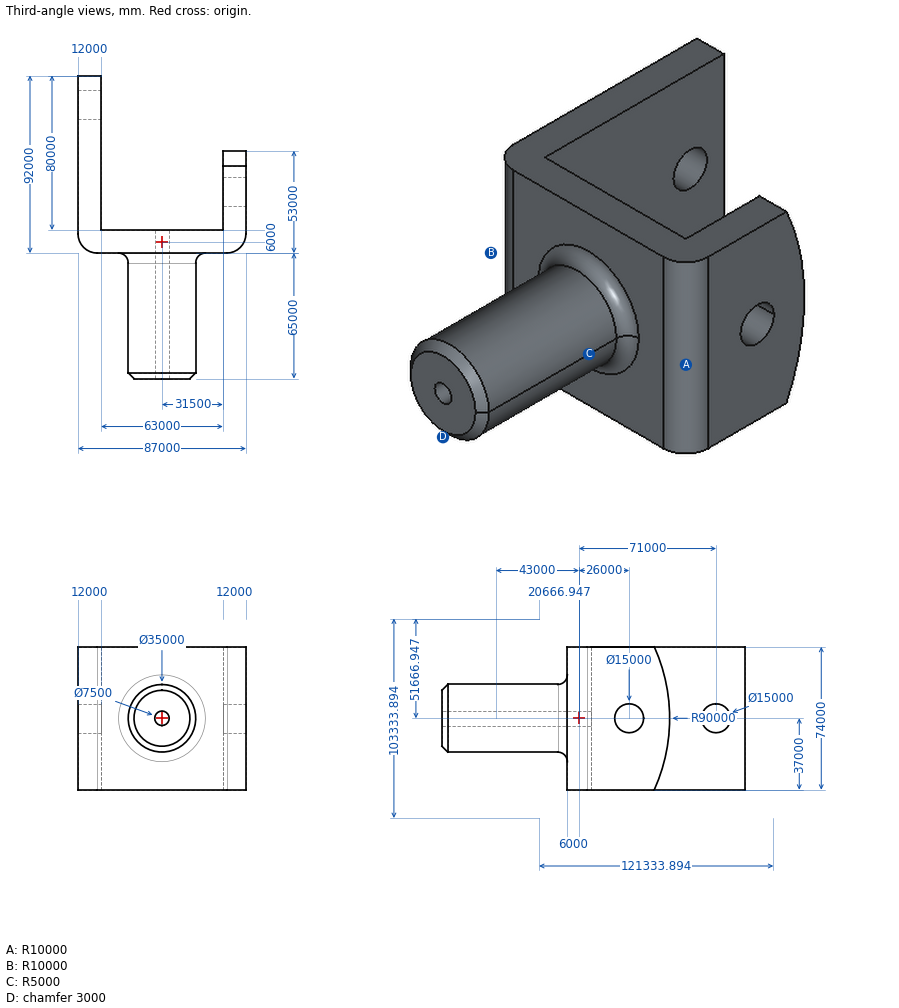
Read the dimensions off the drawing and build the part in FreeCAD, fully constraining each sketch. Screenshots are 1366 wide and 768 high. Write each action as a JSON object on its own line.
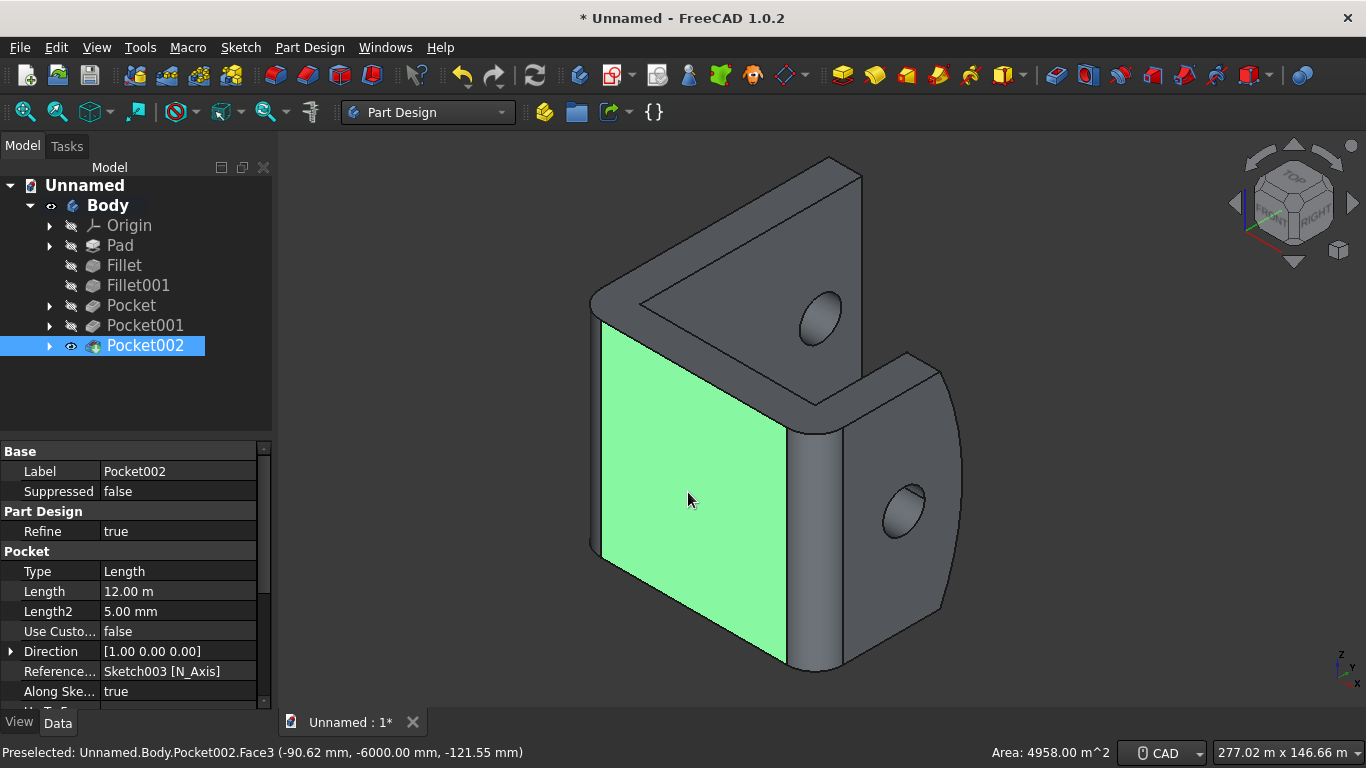
{"action": "left_click", "coordinate": [612, 76]}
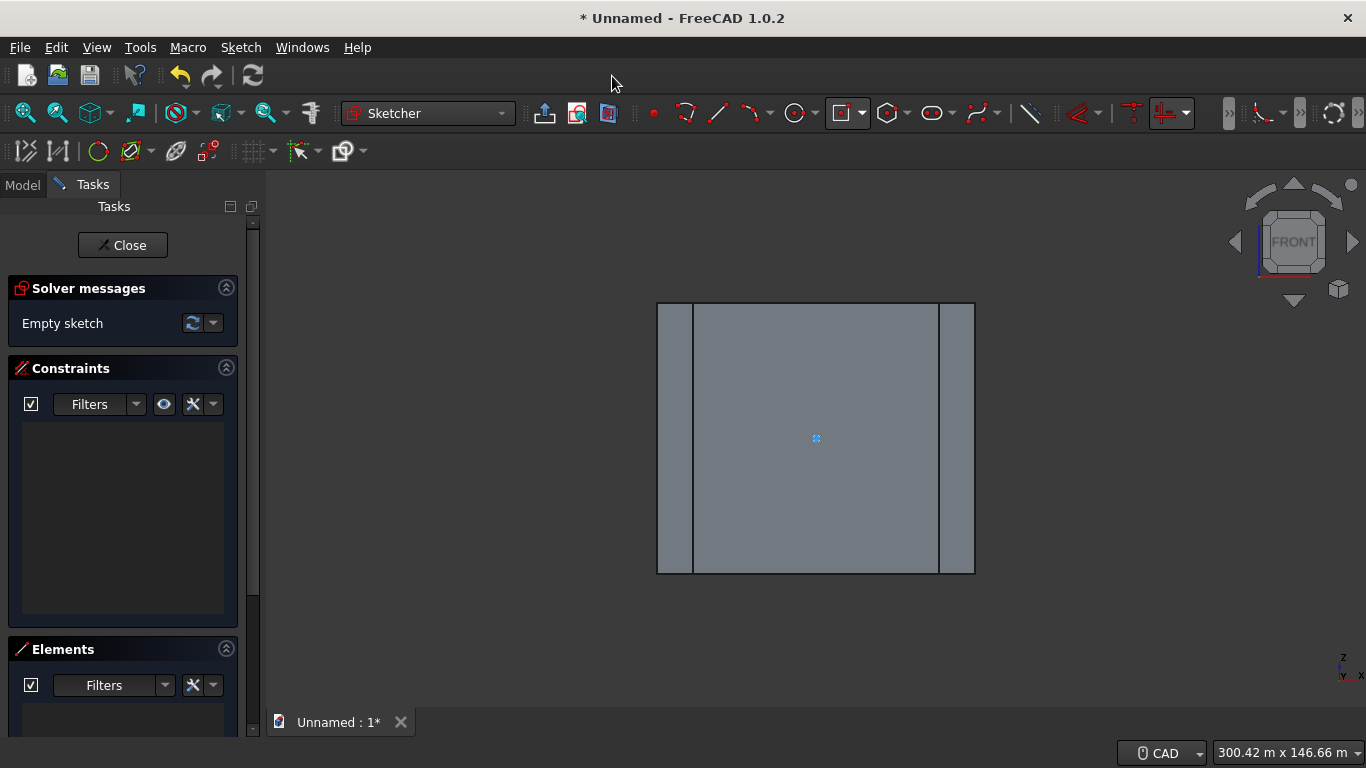
{"action": "scroll", "coordinate": [856, 439], "scroll_direction": "up", "scroll_amount": 5}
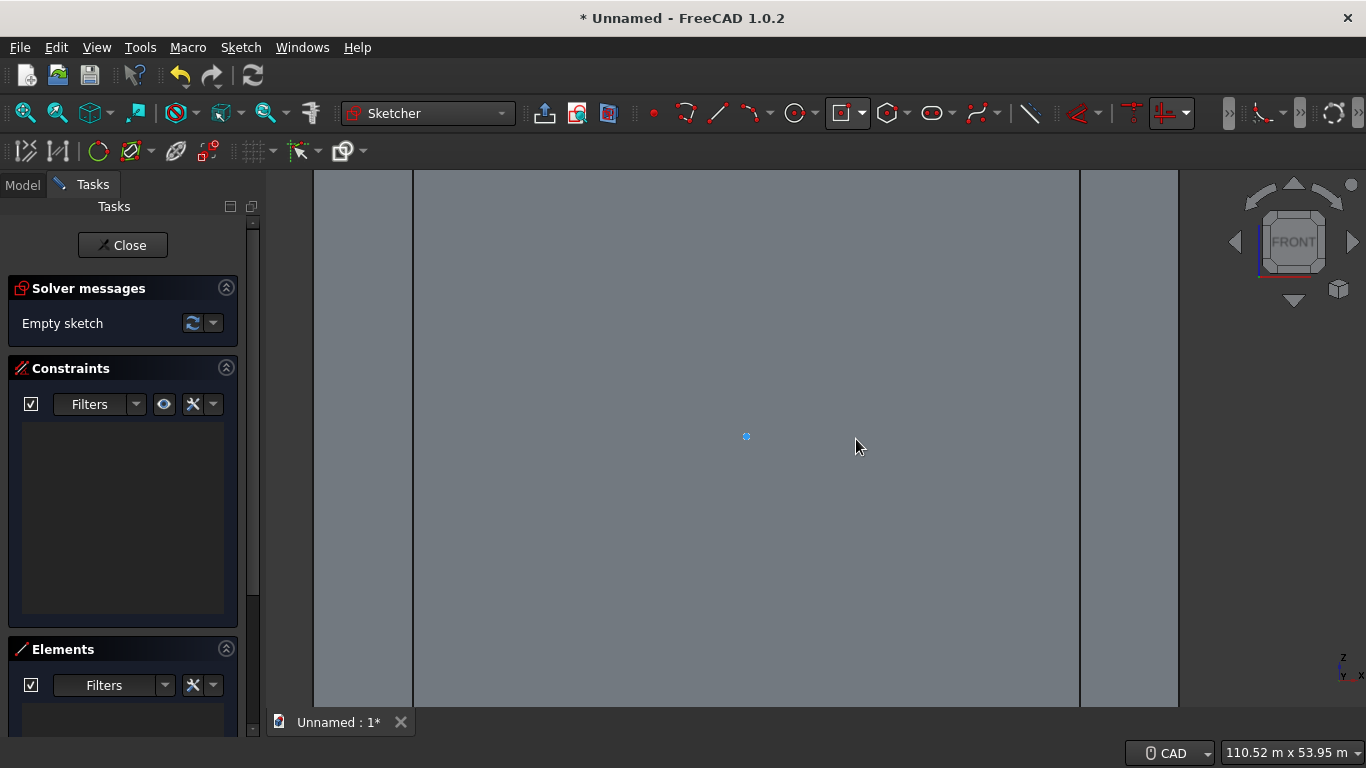
{"action": "left_click", "coordinate": [796, 114]}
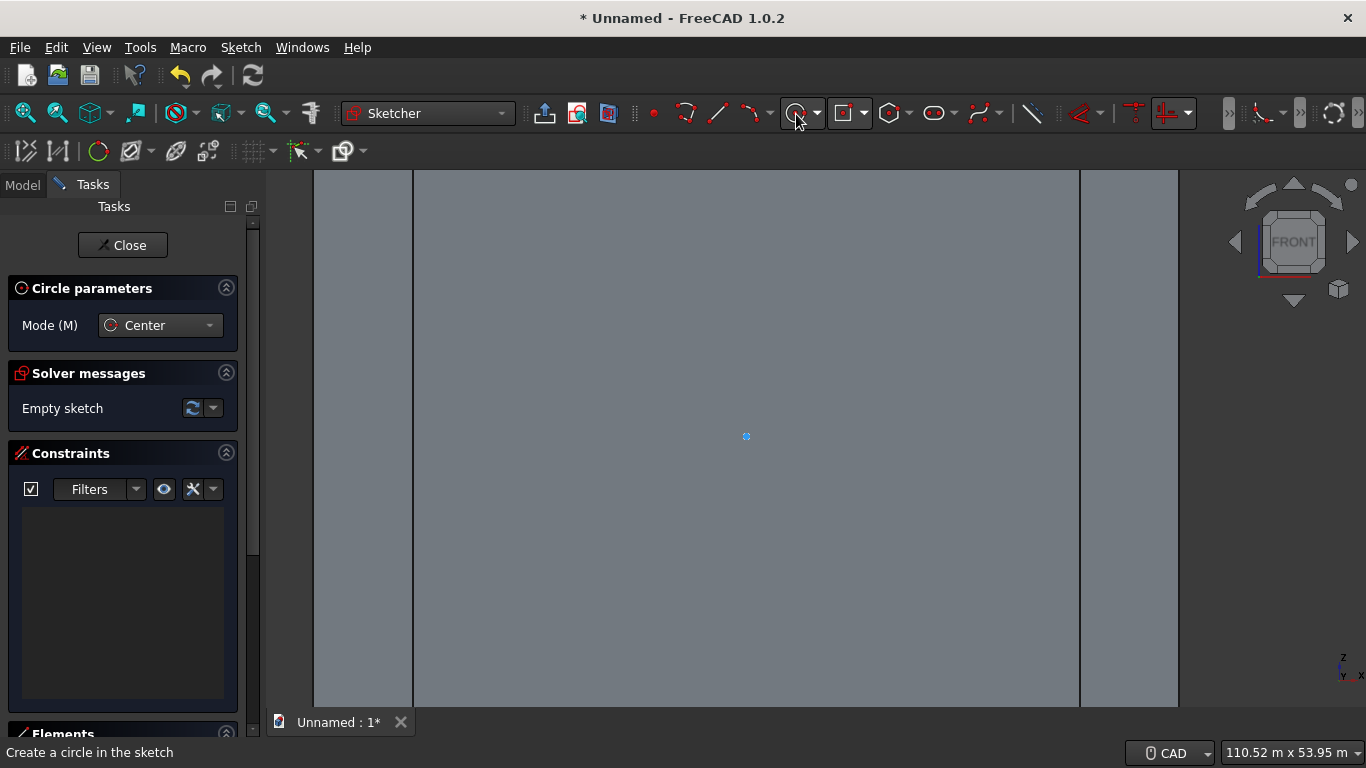
{"action": "left_click", "coordinate": [746, 437]}
{"action": "left_click", "coordinate": [870, 314]}
{"action": "key", "text": "Escape"}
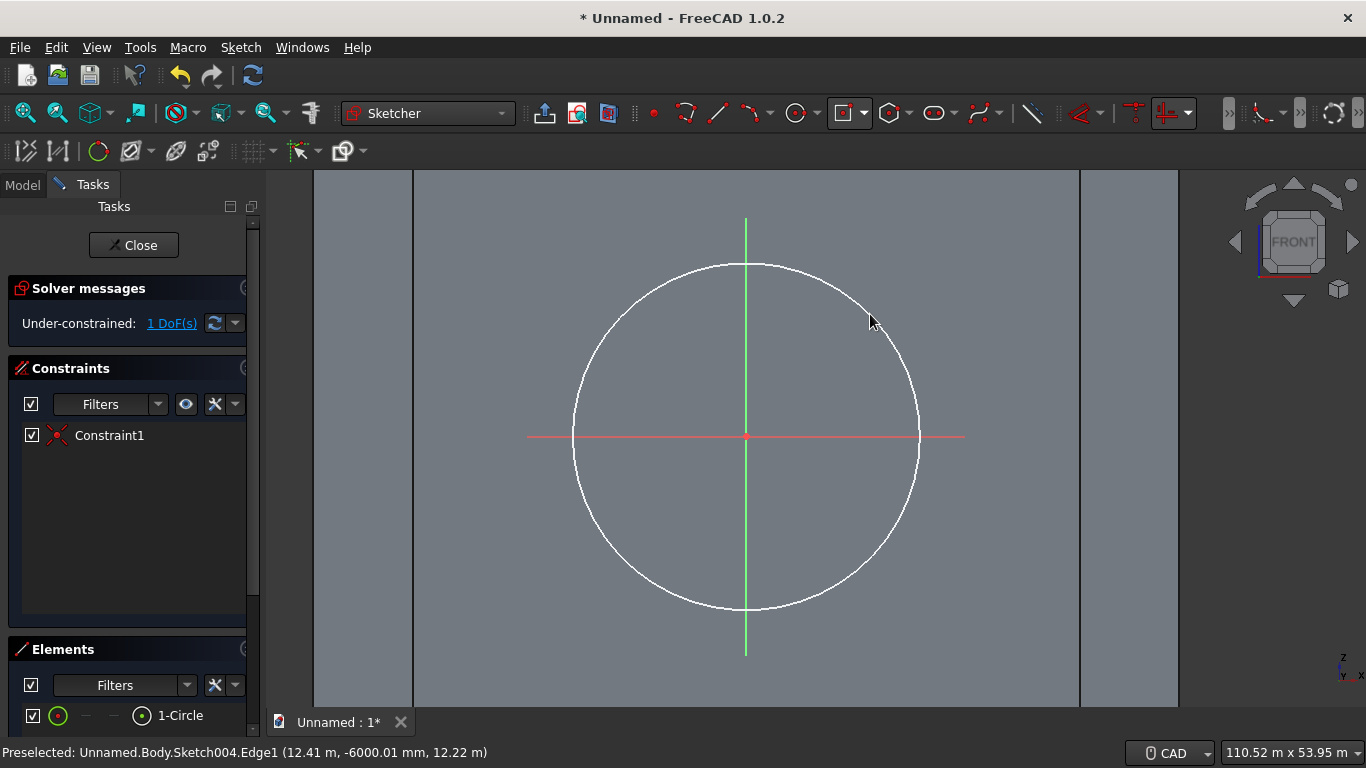
{"action": "left_click", "coordinate": [1080, 114]}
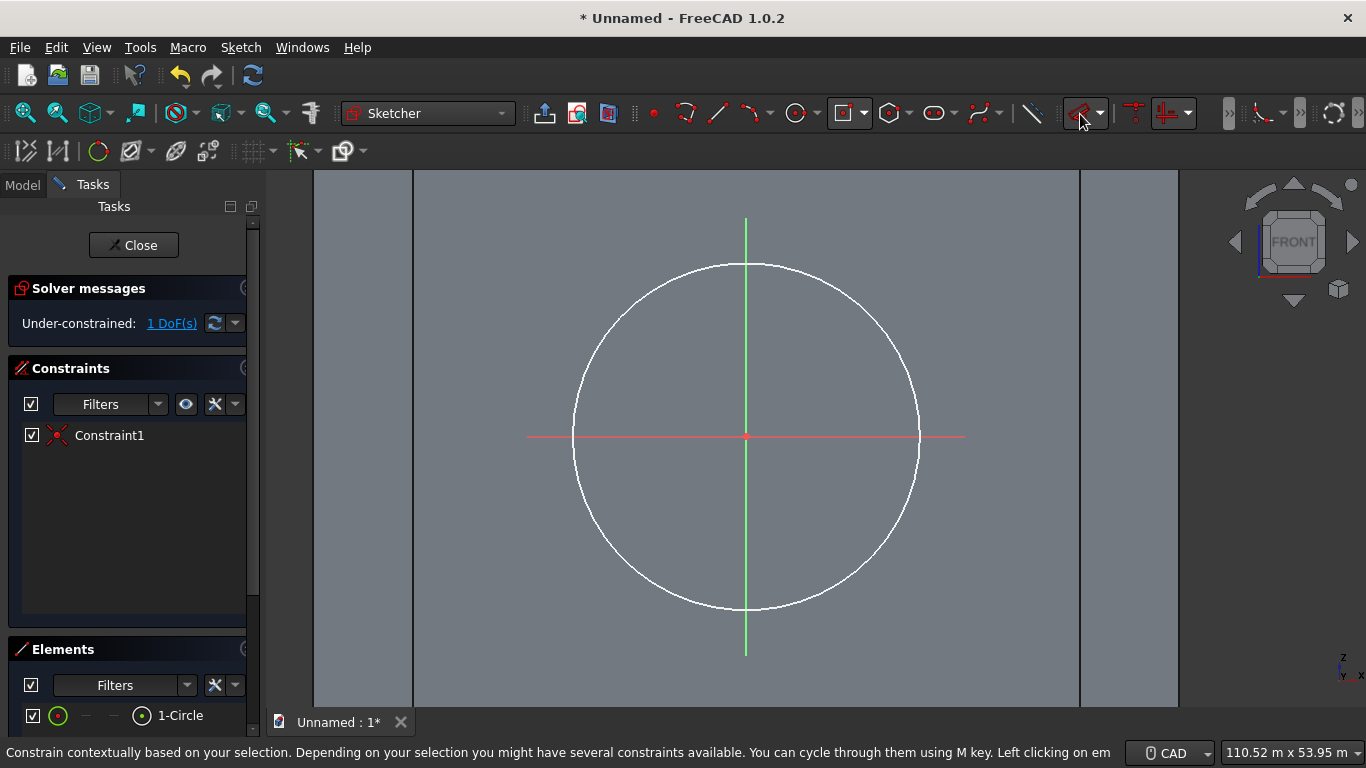
{"action": "left_click", "coordinate": [869, 314]}
{"action": "left_click", "coordinate": [892, 291]}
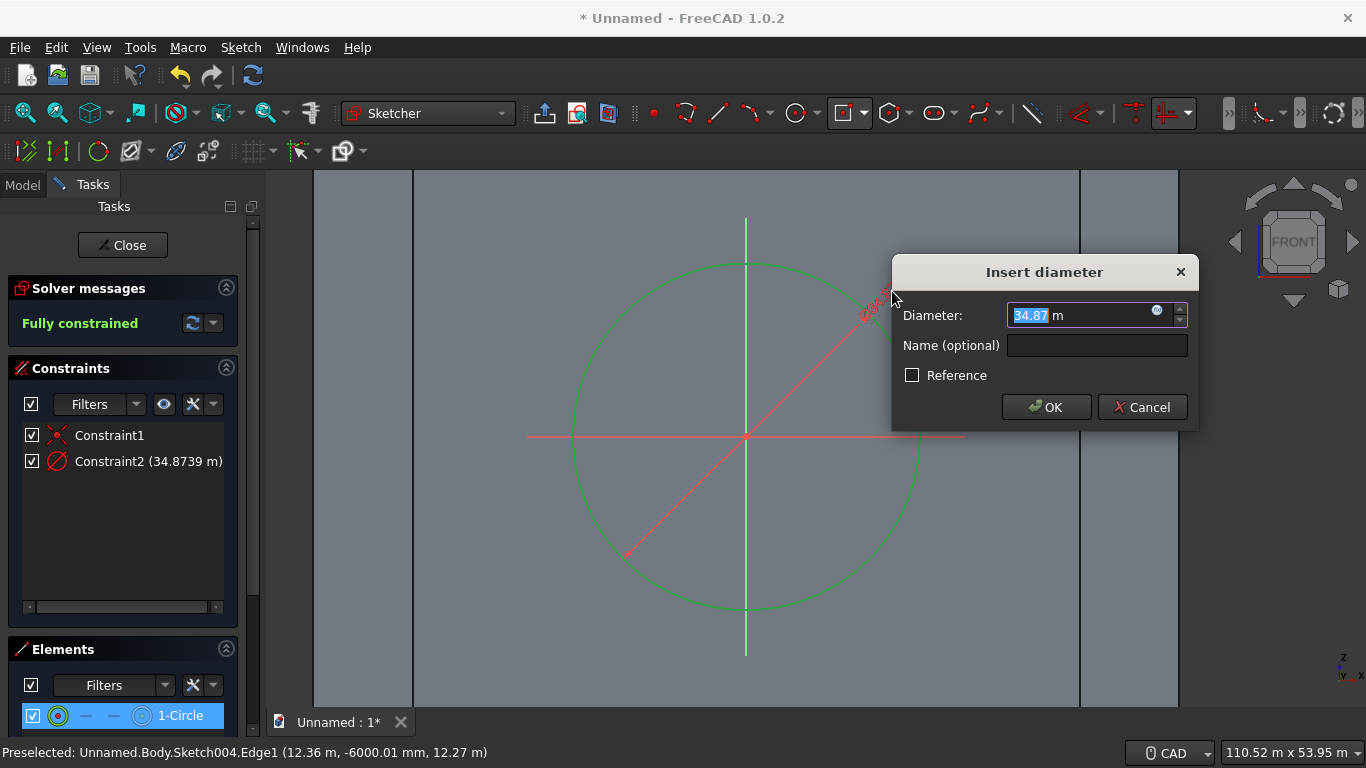
{"action": "key", "text": "ctrl+a"}
{"action": "type", "text": "35000 mm"}
{"action": "key", "text": "Return"}
{"action": "key", "text": "Escape"}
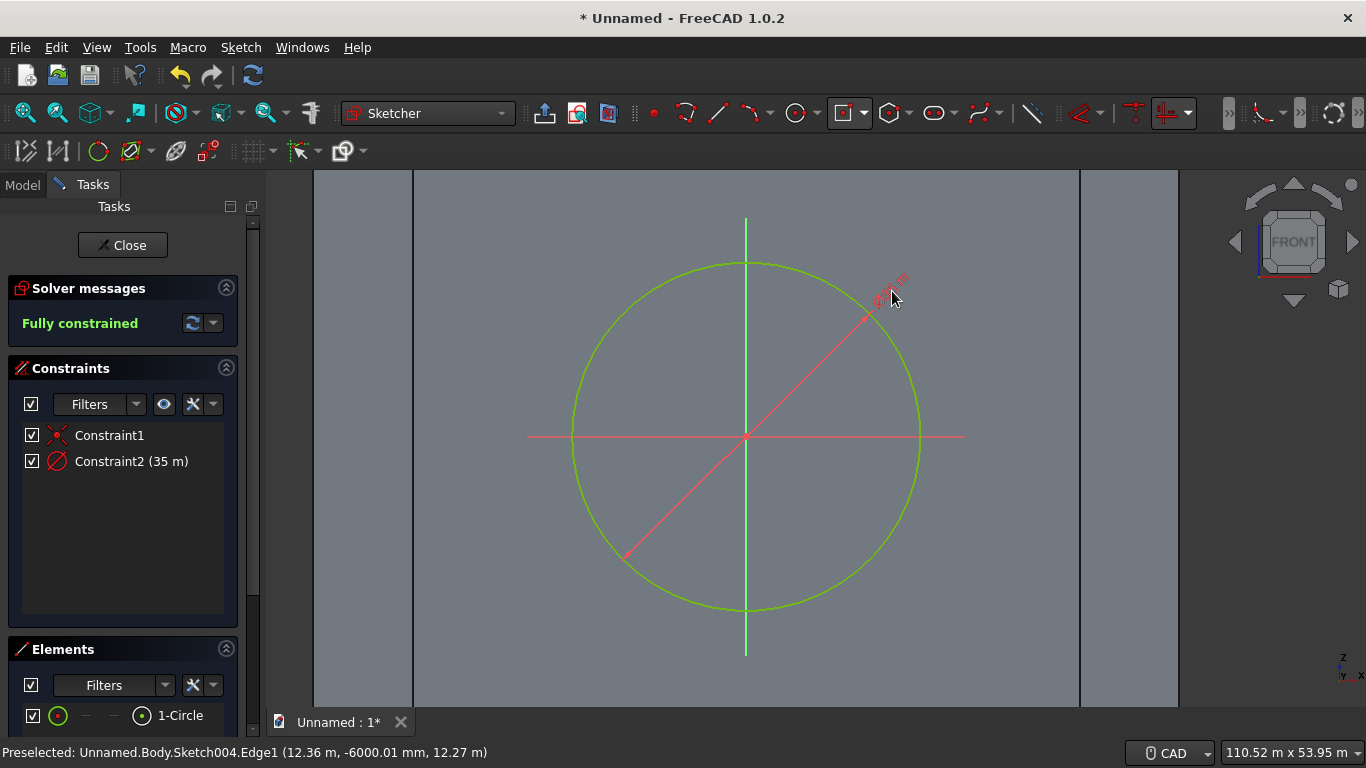
{"action": "left_click", "coordinate": [123, 245]}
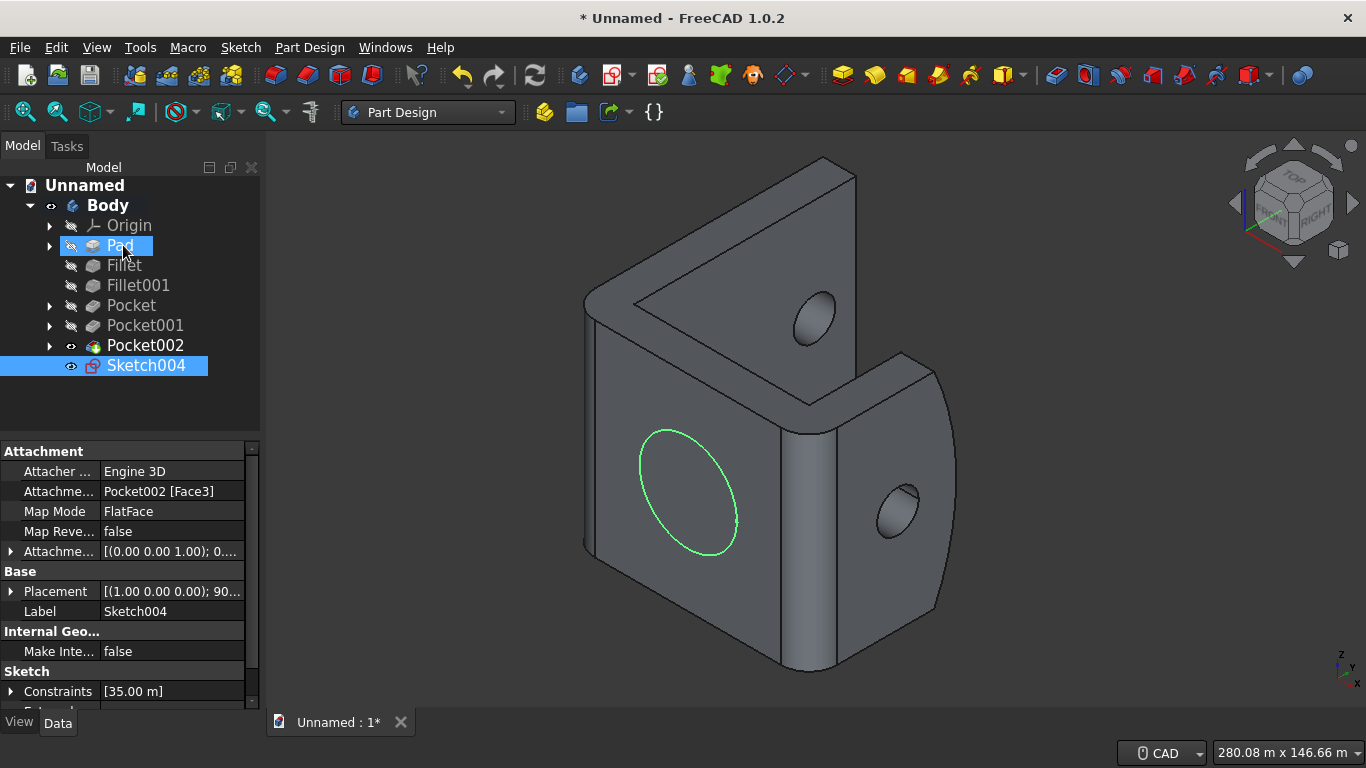
{"action": "left_click", "coordinate": [844, 76]}